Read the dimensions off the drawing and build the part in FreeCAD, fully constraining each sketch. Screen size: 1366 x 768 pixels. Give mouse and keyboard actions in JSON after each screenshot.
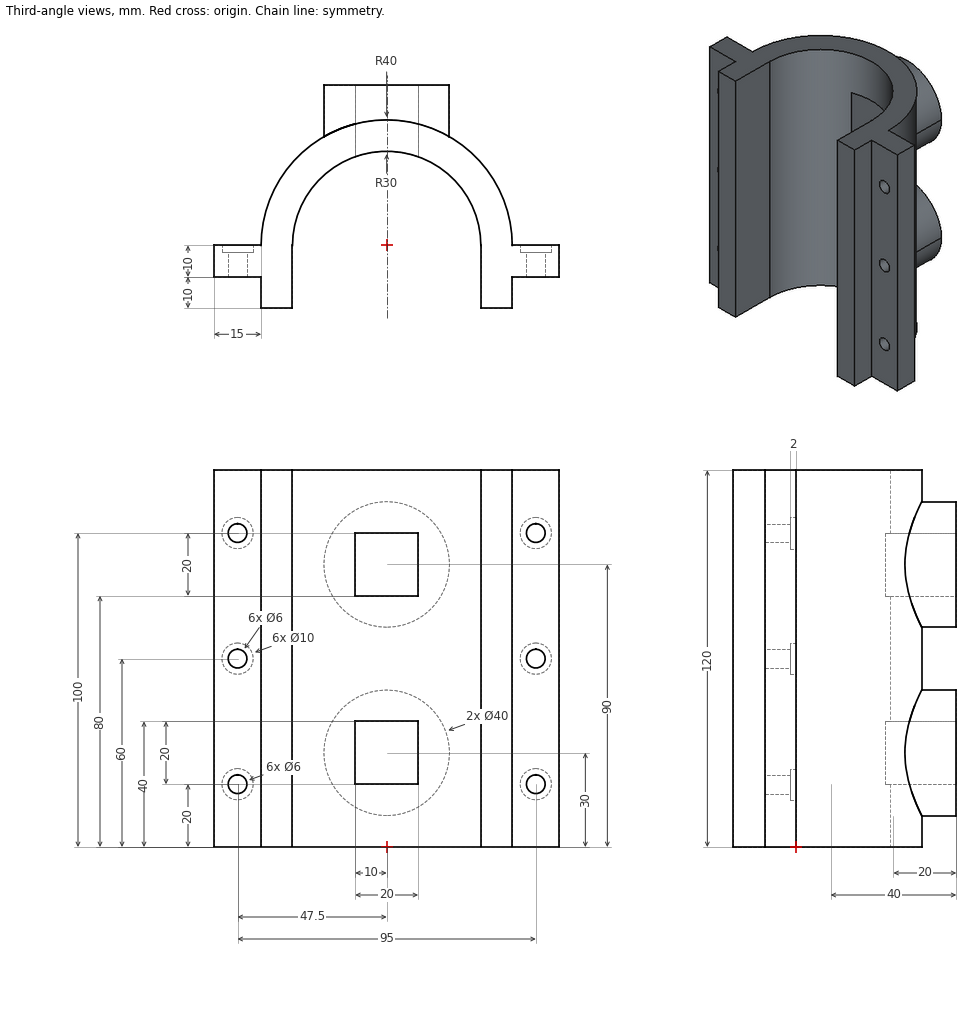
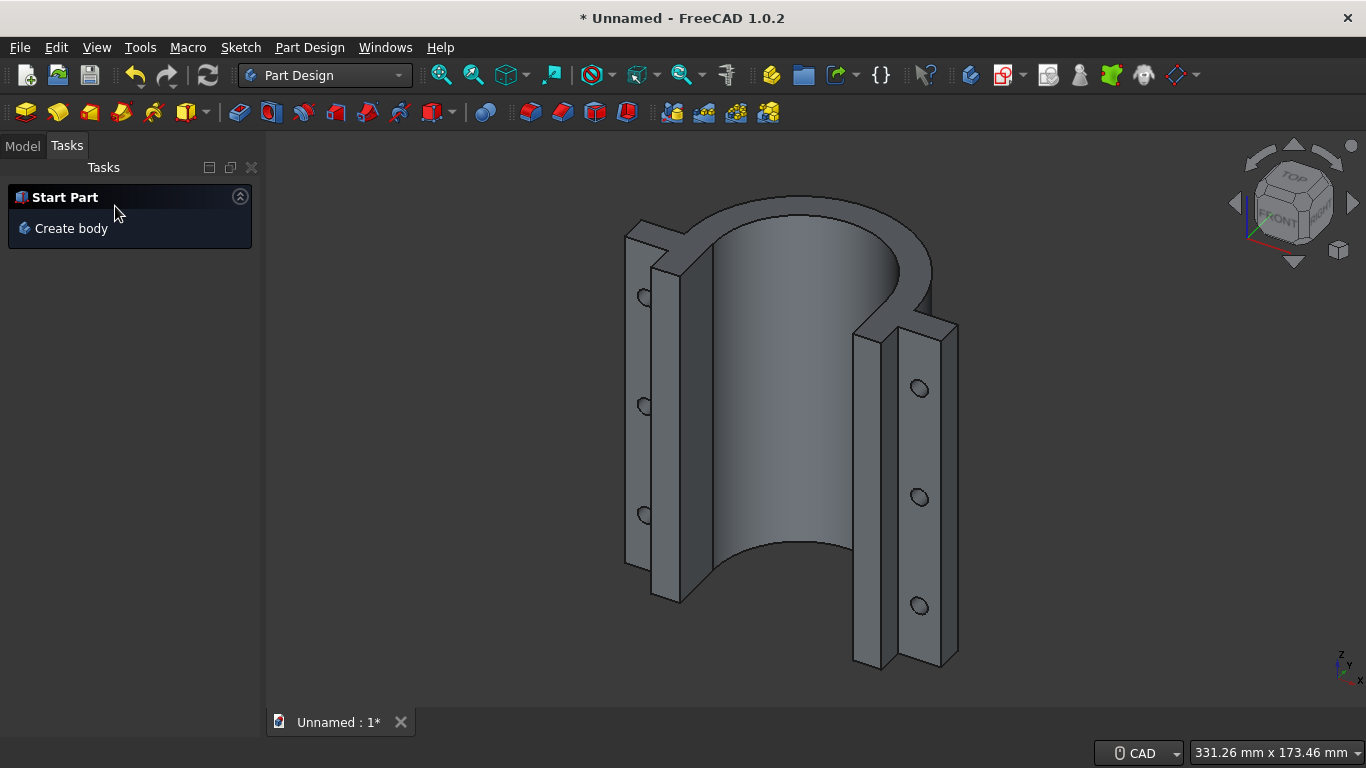
{"action": "key", "text": "4"}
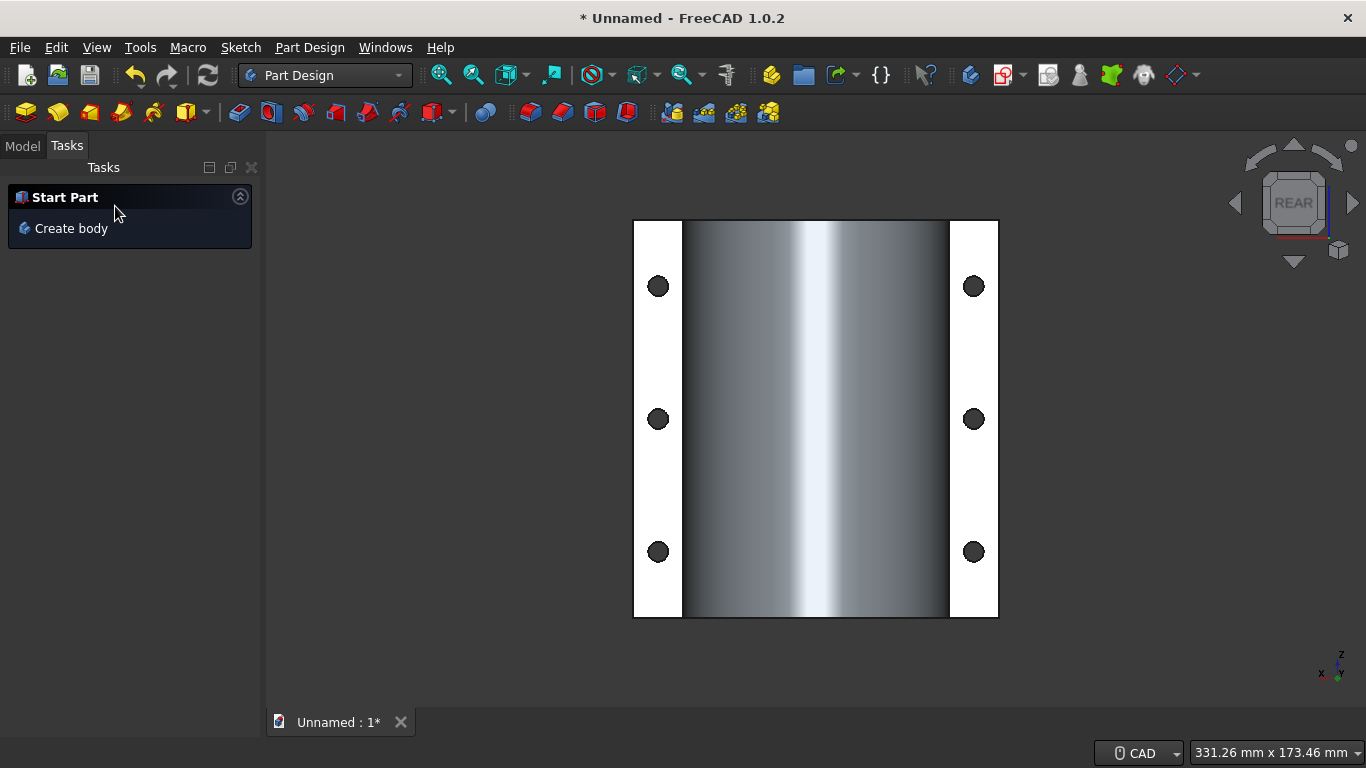
{"action": "left_click", "coordinate": [658, 247]}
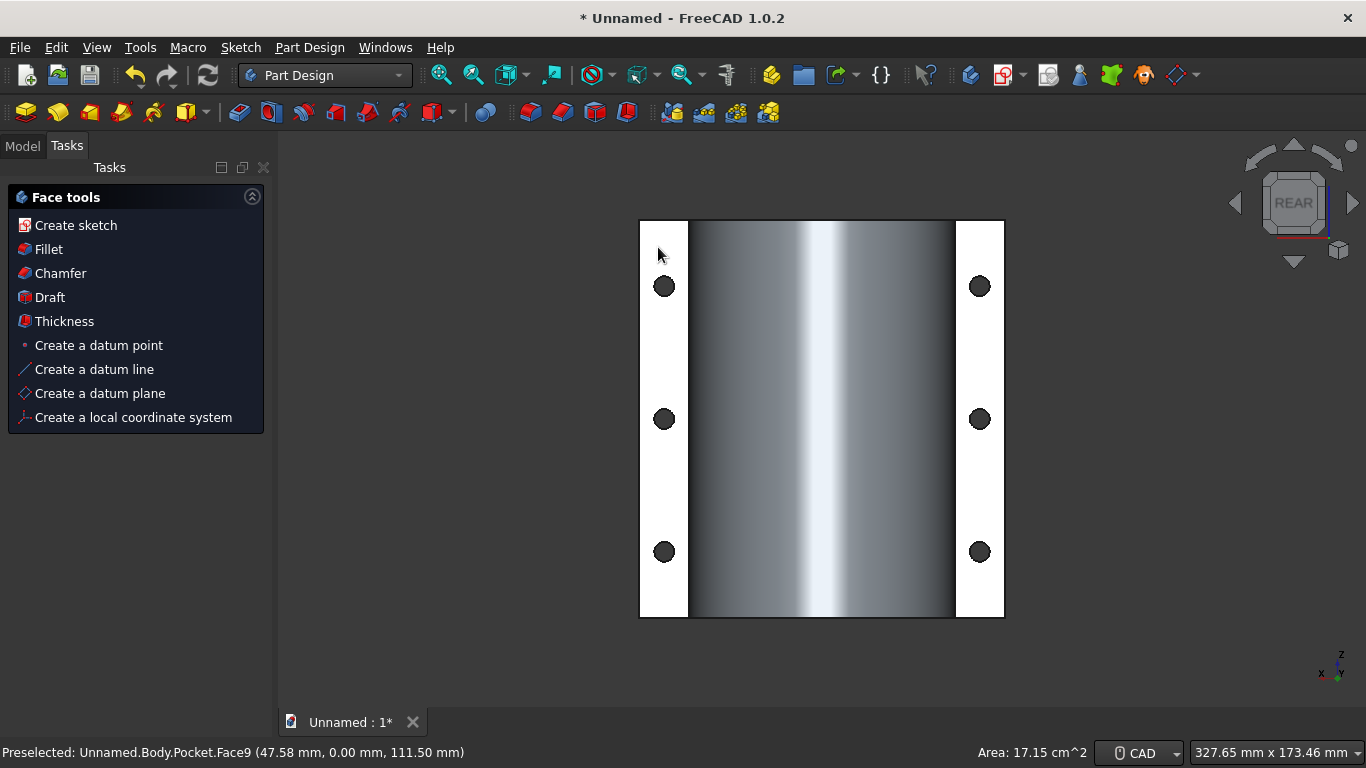
{"action": "left_click", "coordinate": [1004, 76]}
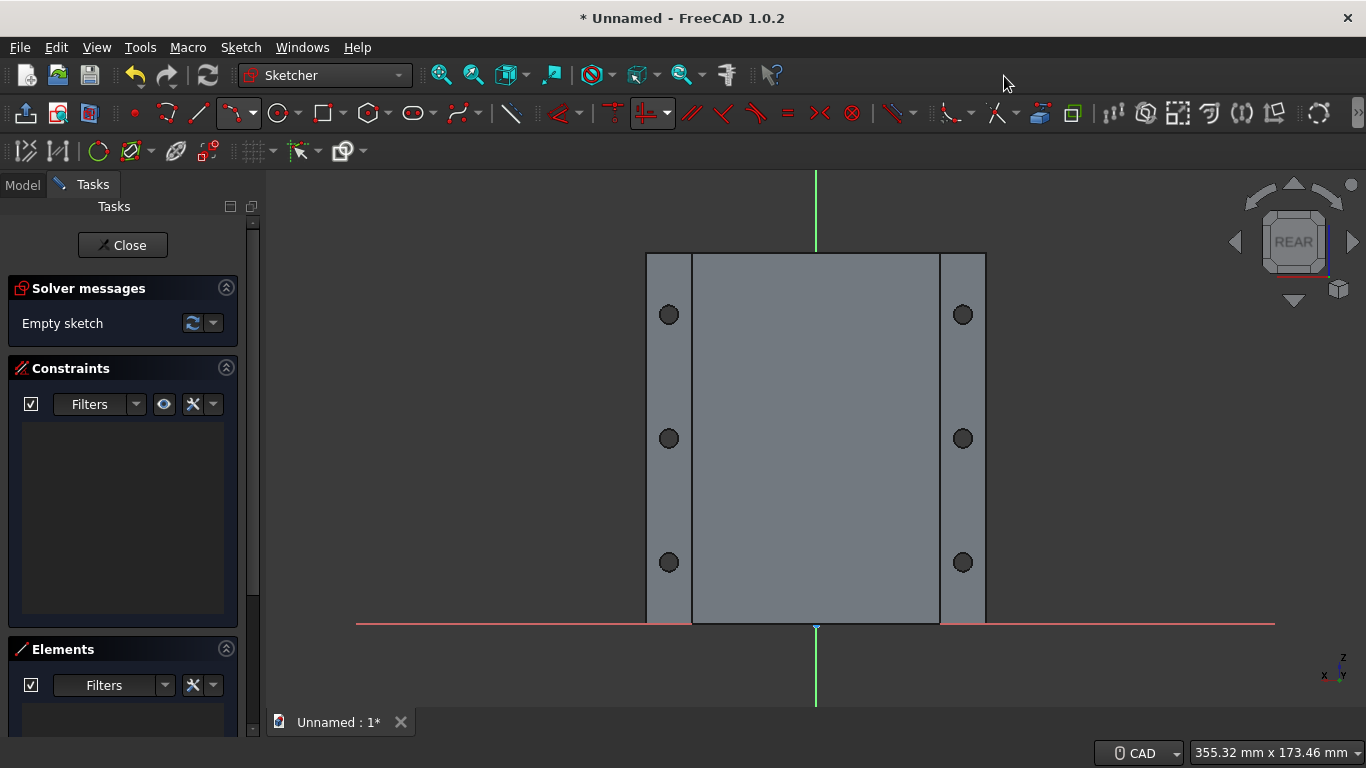
{"action": "left_click", "coordinate": [90, 114]}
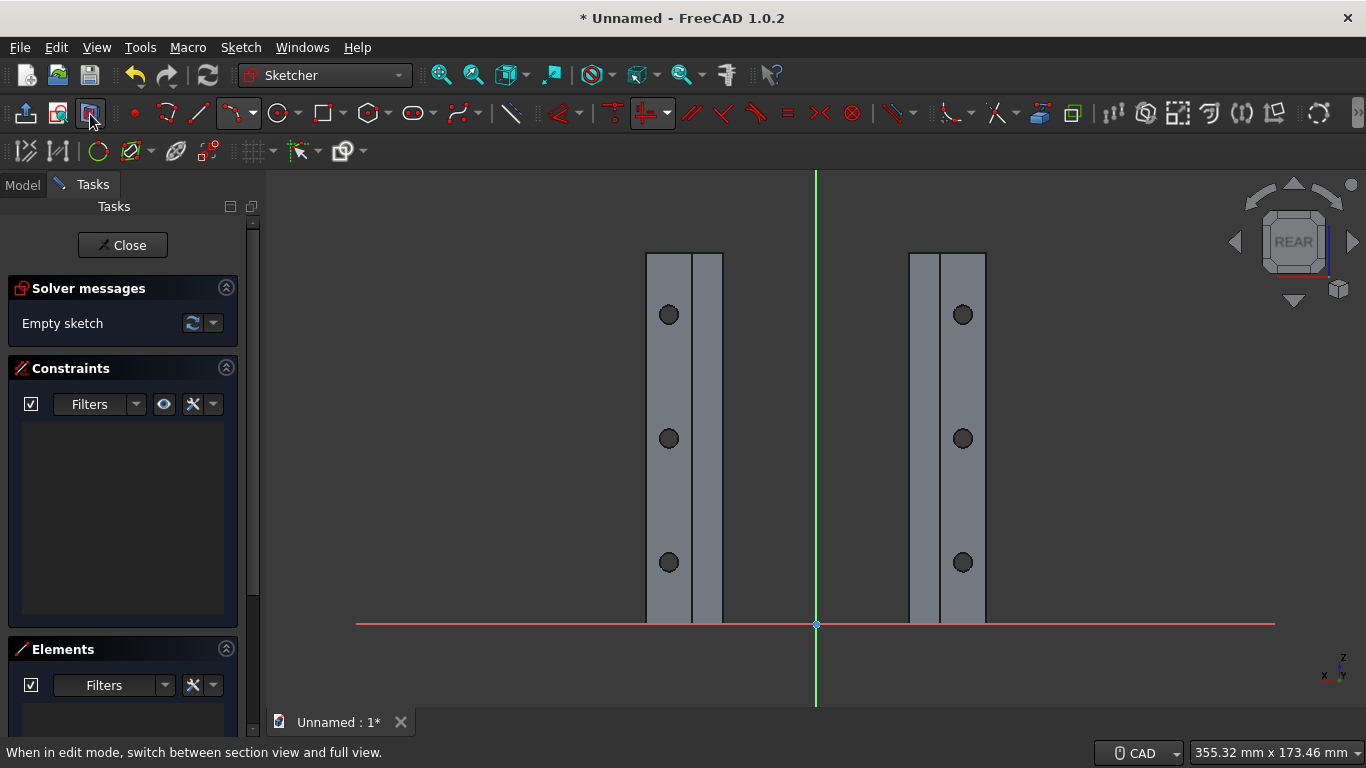
{"action": "left_click", "coordinate": [278, 114]}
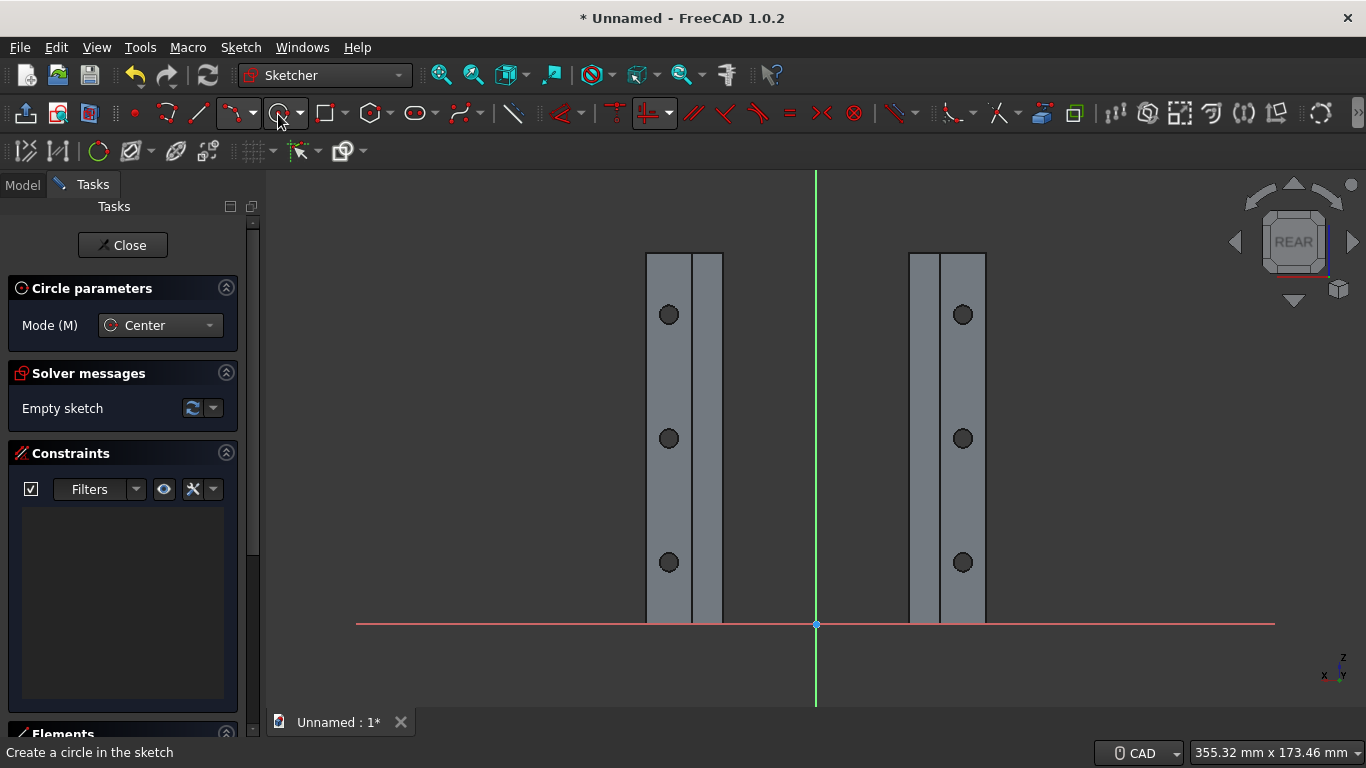
{"action": "scroll", "coordinate": [963, 438], "scroll_direction": "up", "scroll_amount": 2}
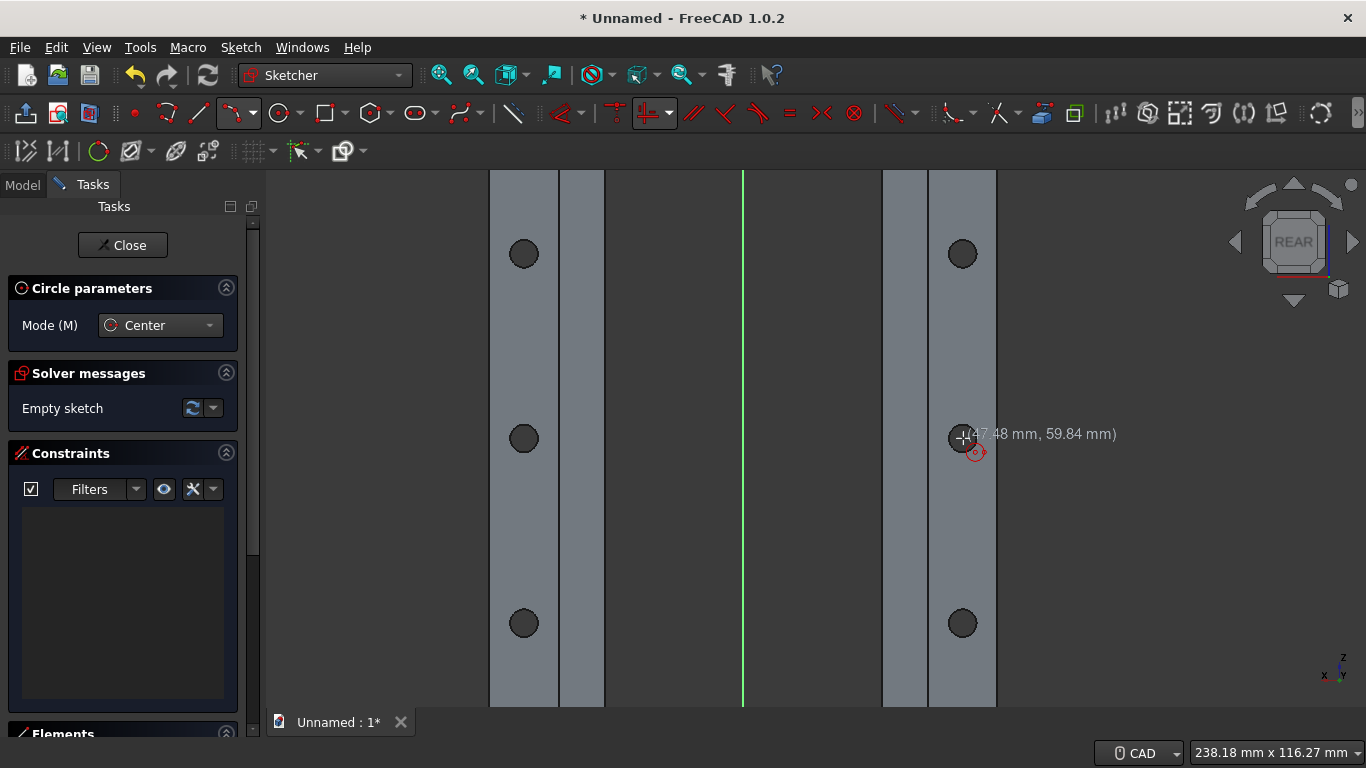
{"action": "left_click", "coordinate": [963, 438]}
{"action": "left_click", "coordinate": [979, 422]}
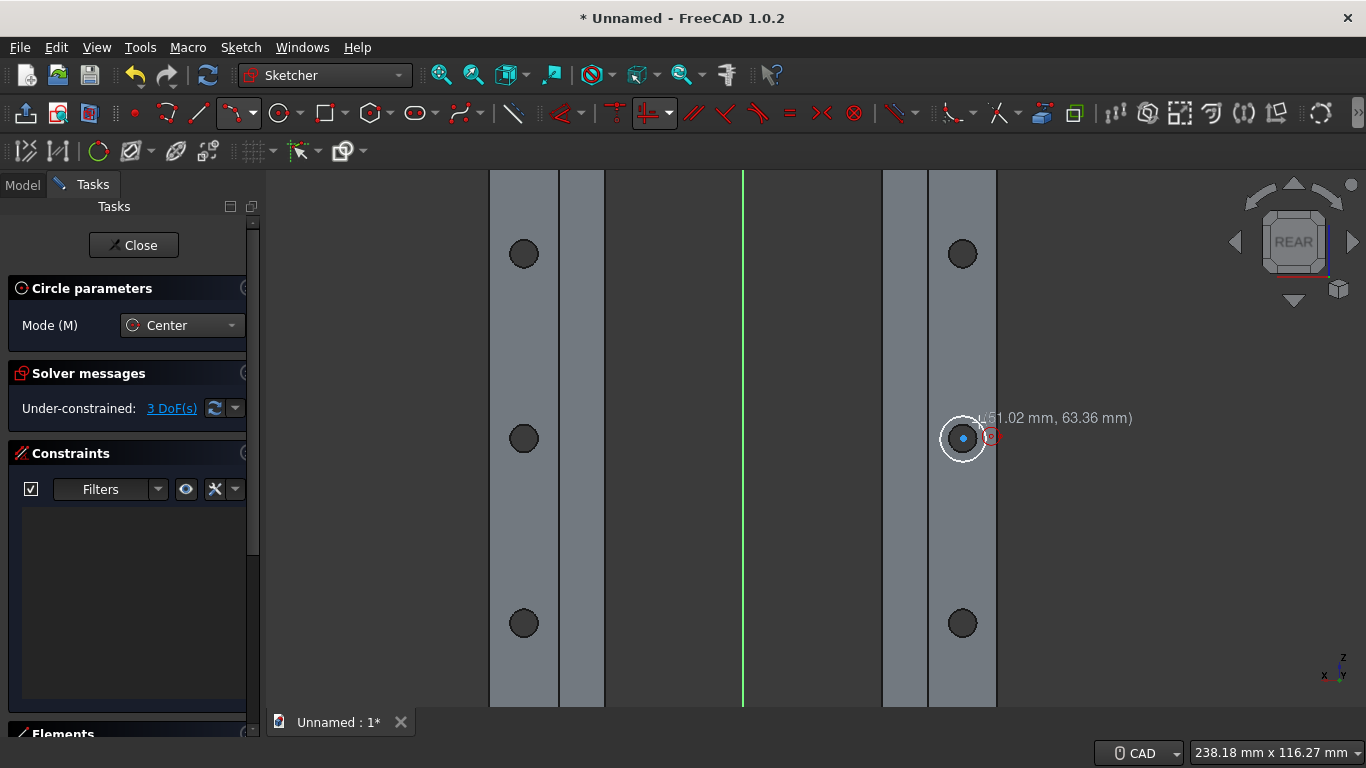
{"action": "left_click", "coordinate": [963, 254]}
{"action": "left_click", "coordinate": [979, 237]}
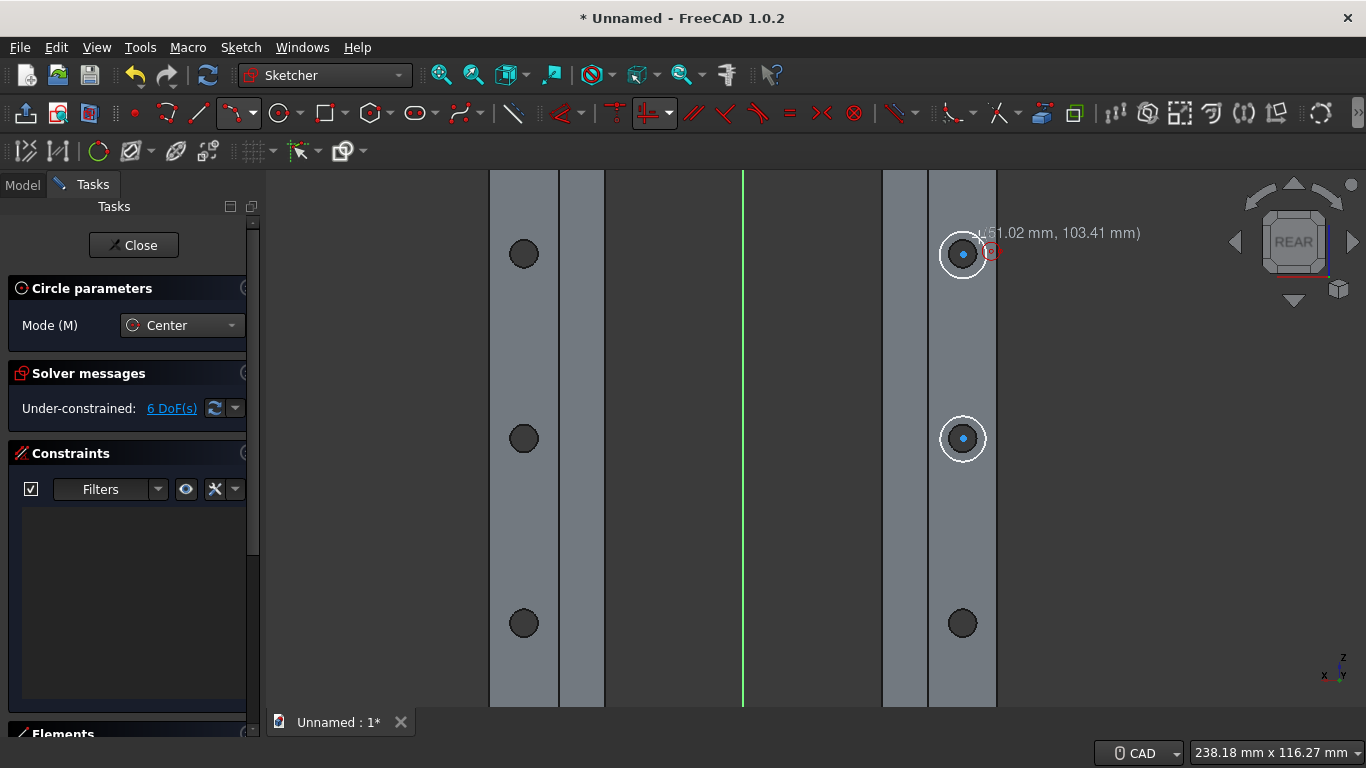
{"action": "left_click", "coordinate": [963, 623]}
{"action": "left_click", "coordinate": [979, 607]}